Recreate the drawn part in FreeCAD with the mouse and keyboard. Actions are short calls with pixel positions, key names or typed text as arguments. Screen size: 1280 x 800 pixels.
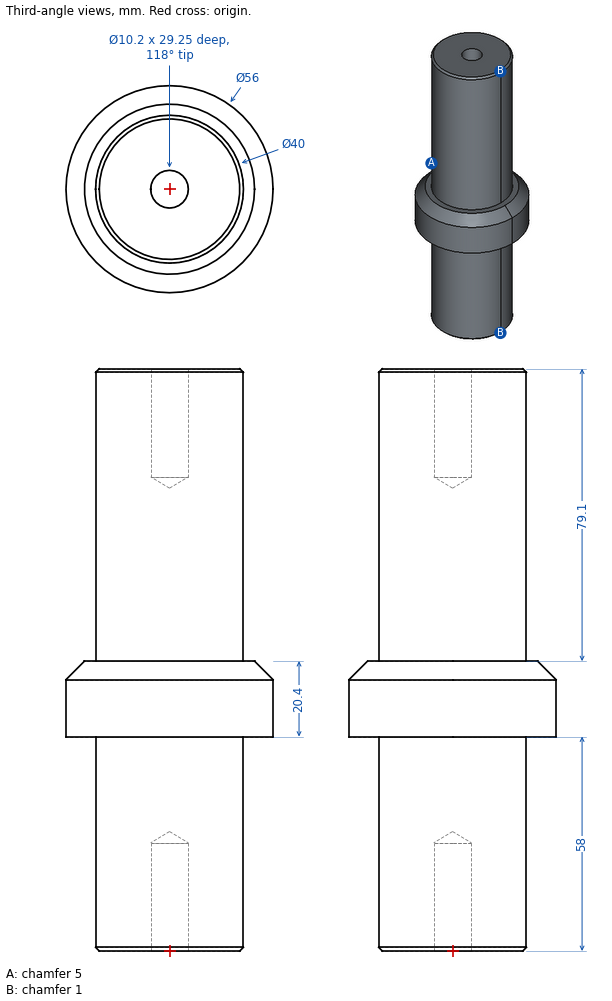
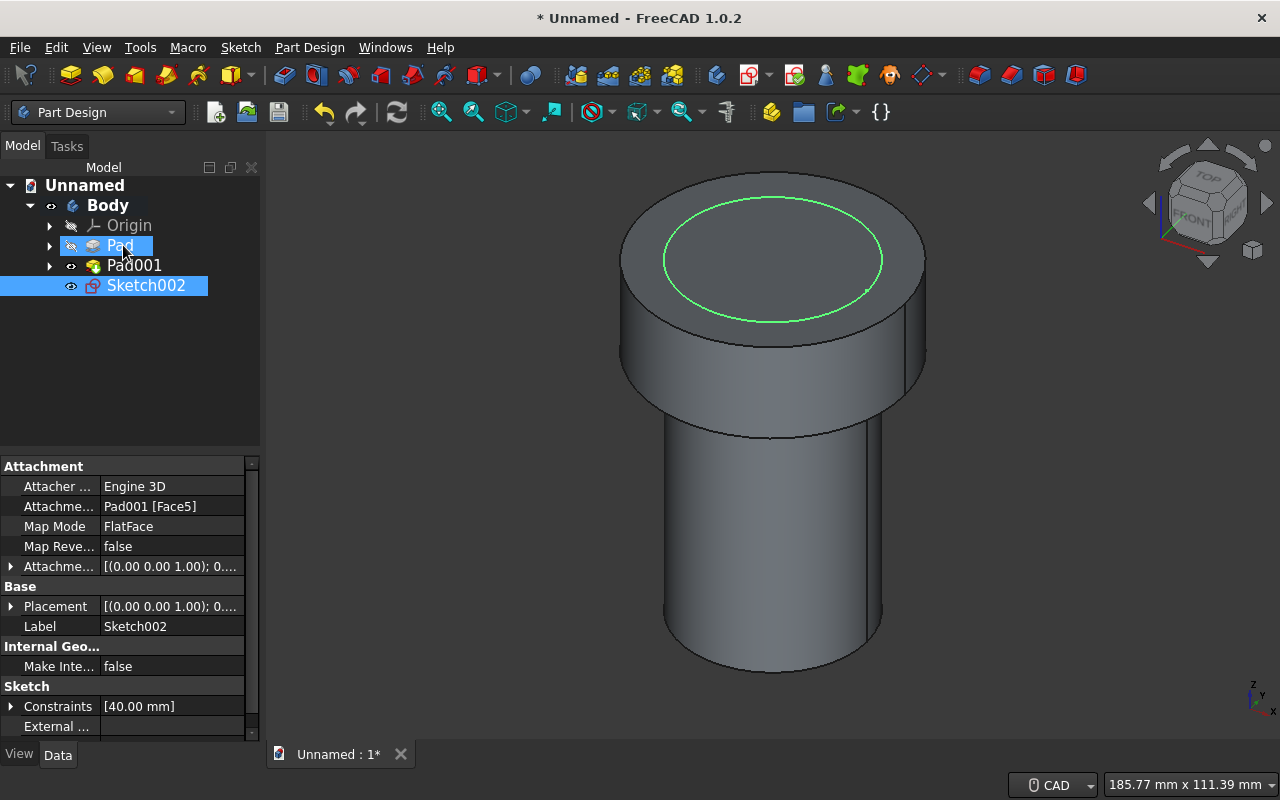
click(72, 76)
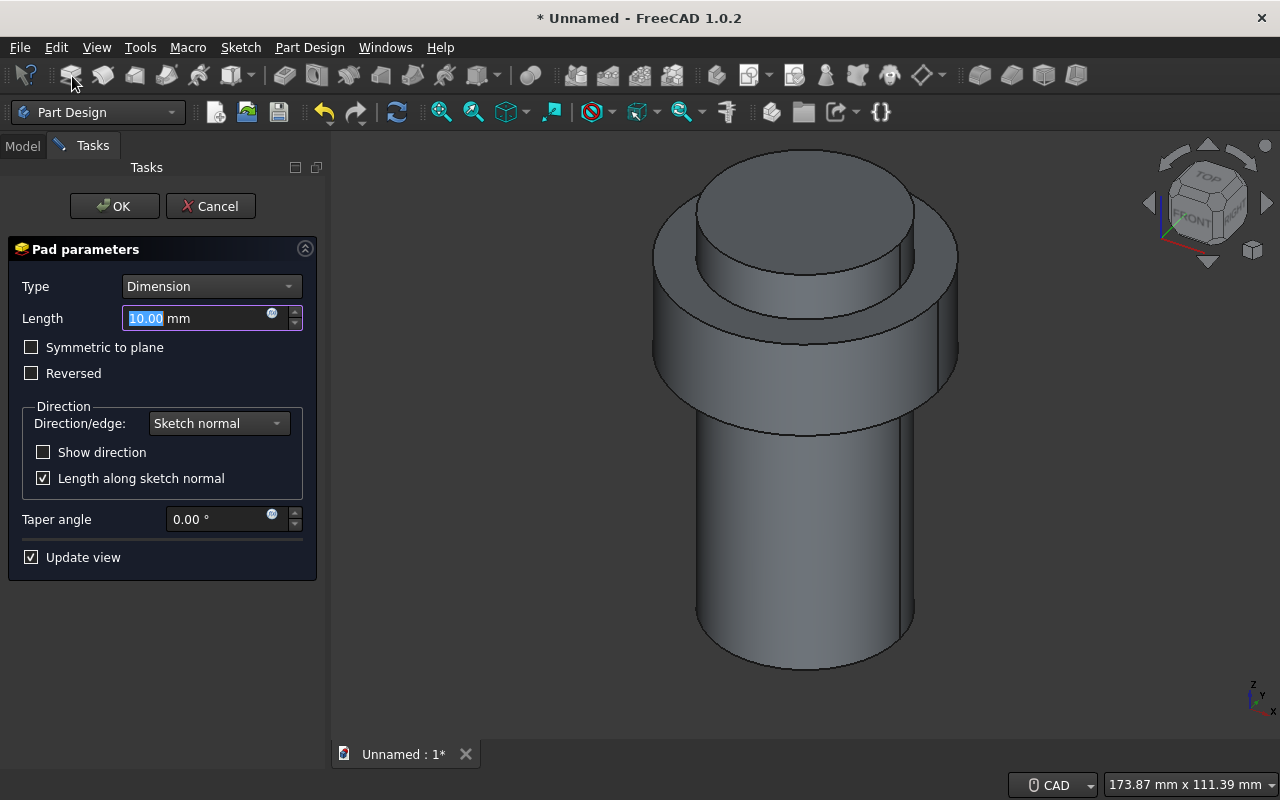
text(79.1)
key(Tab)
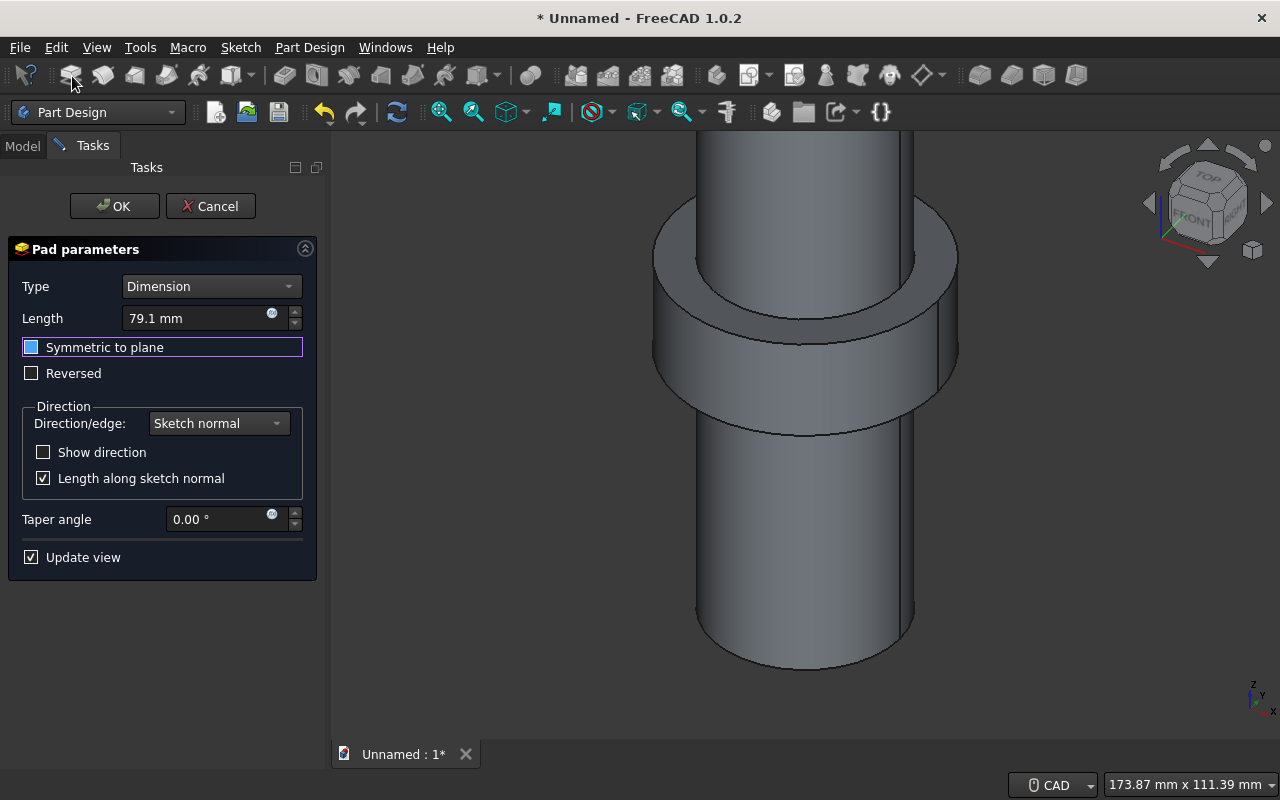
click(115, 206)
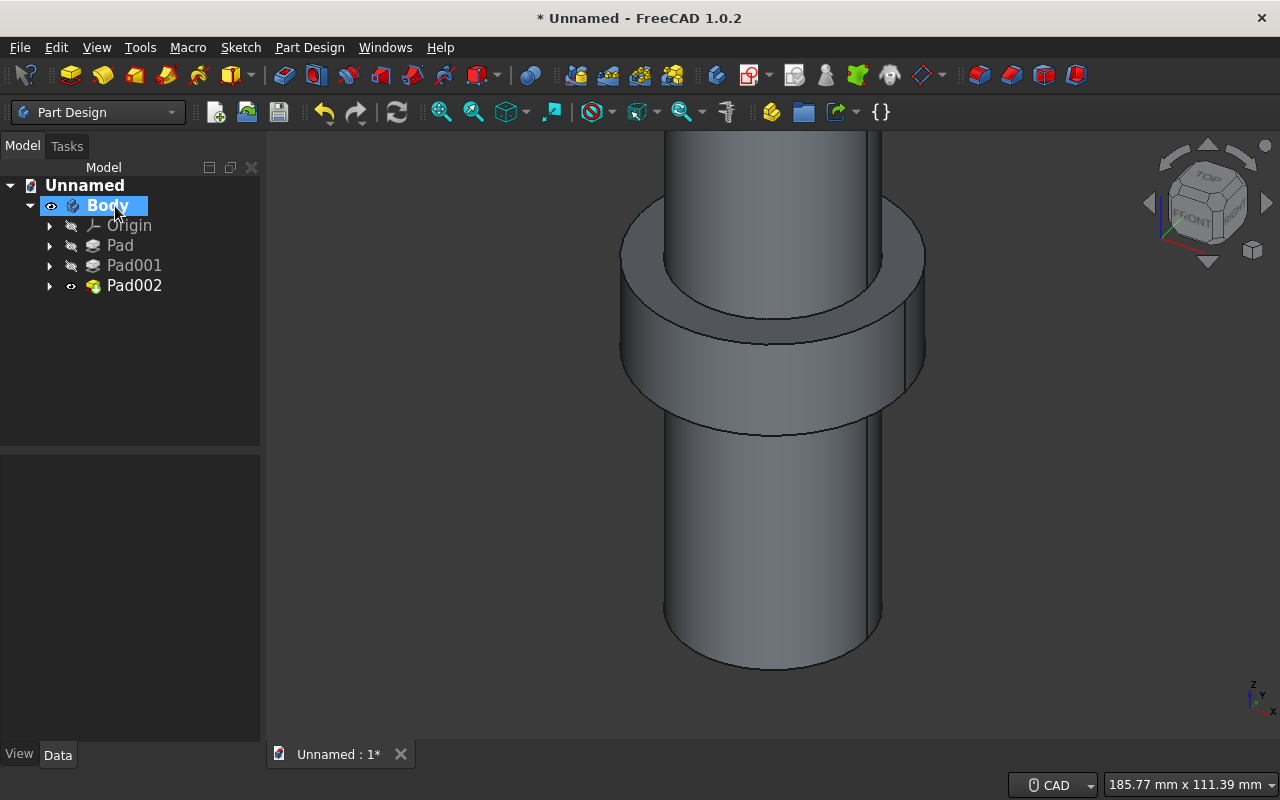
click(442, 112)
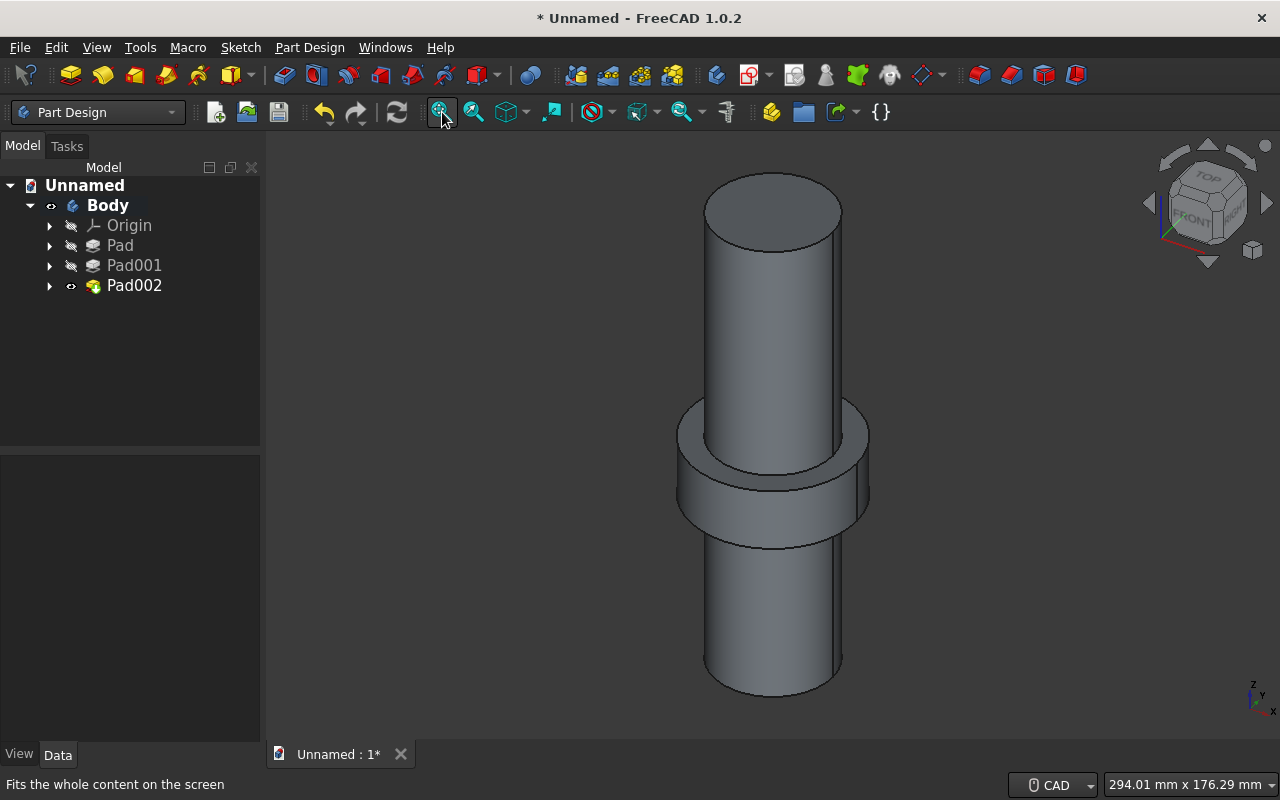
click(677, 441)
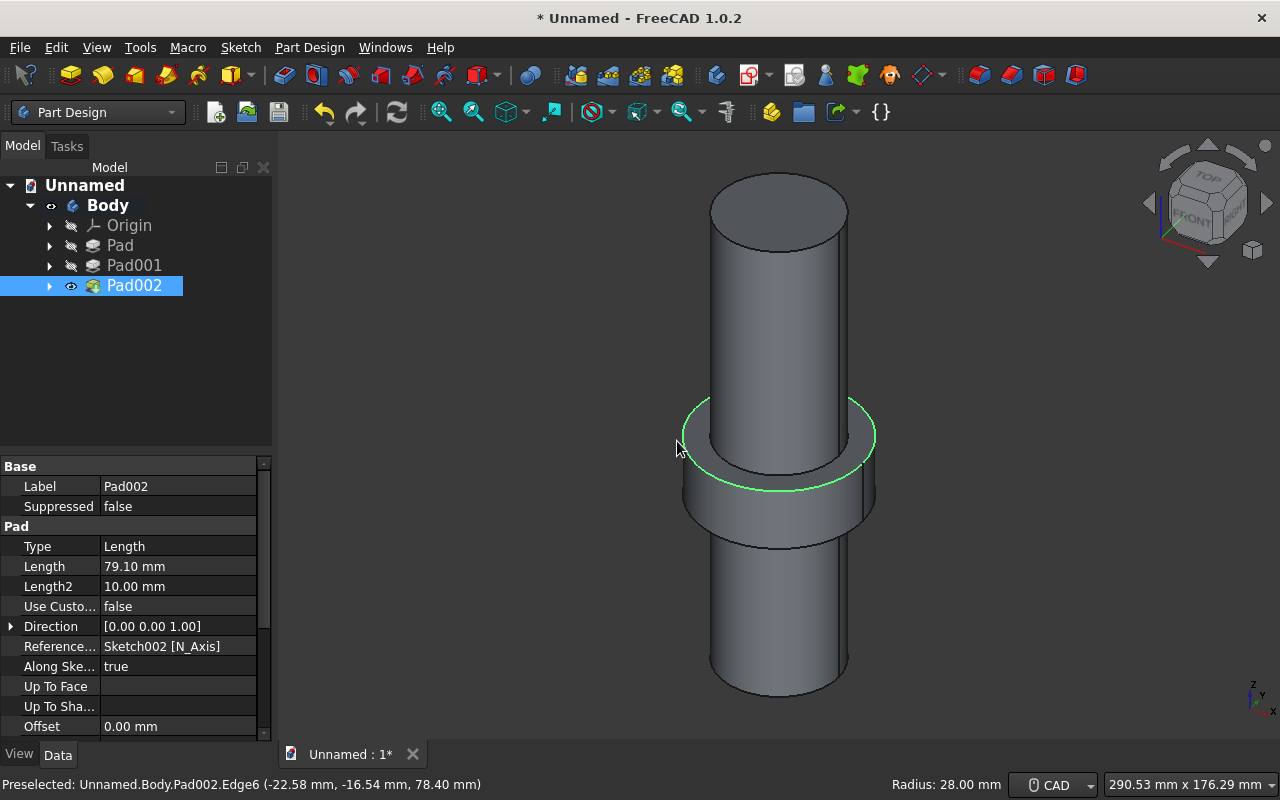
click(1012, 76)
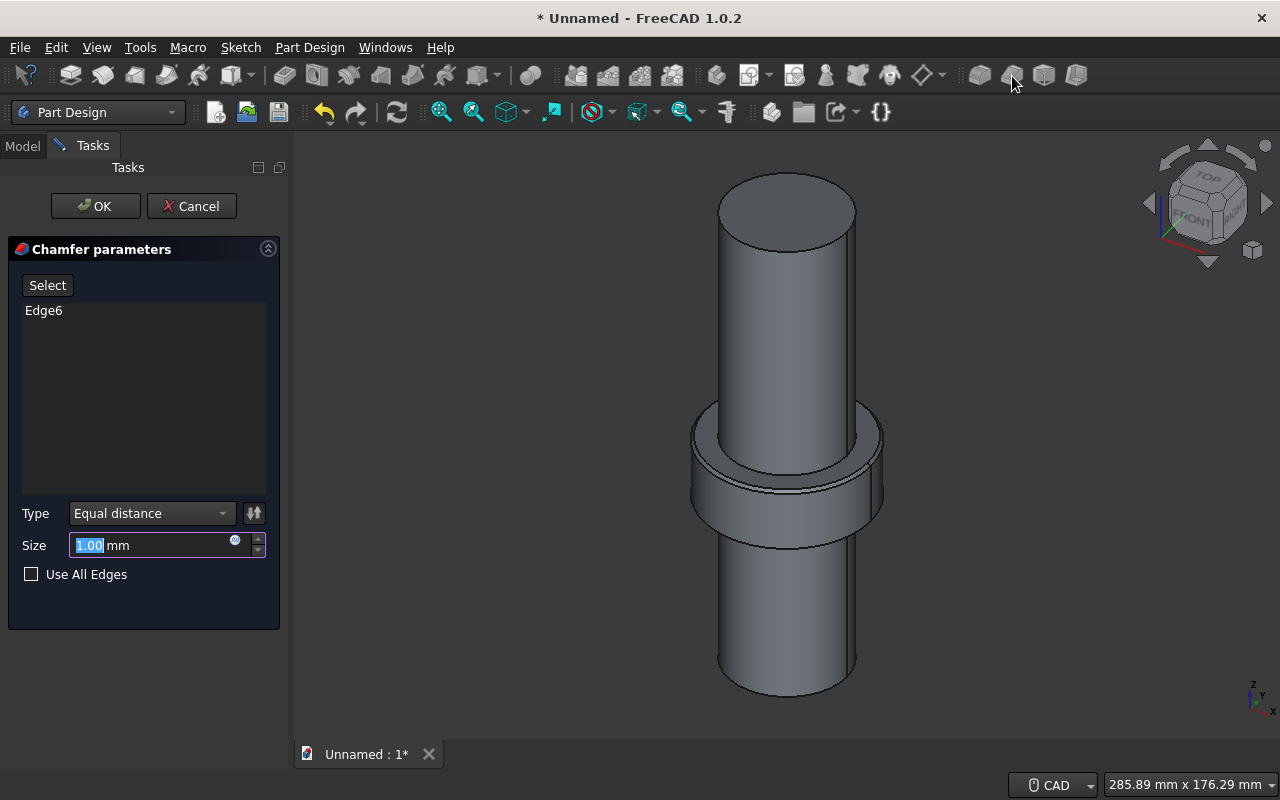
text(5)
key(Tab)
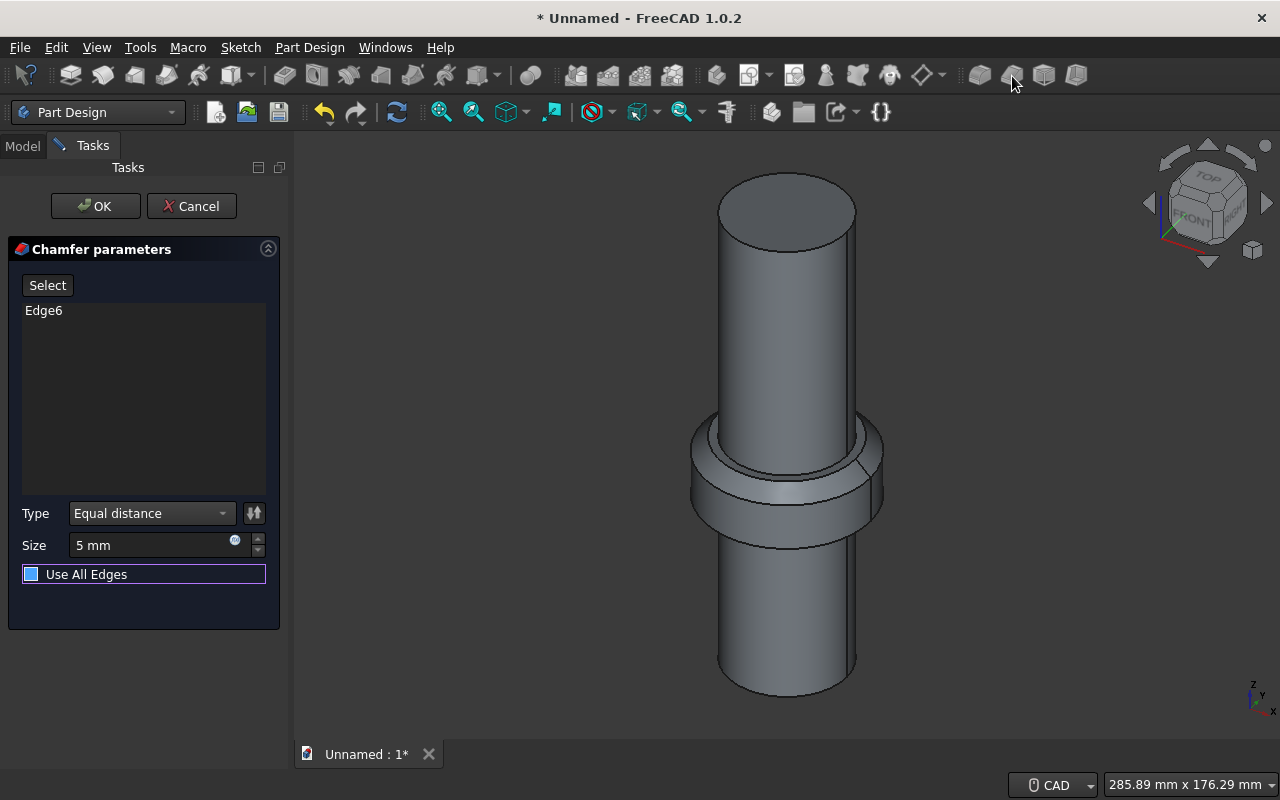
click(96, 206)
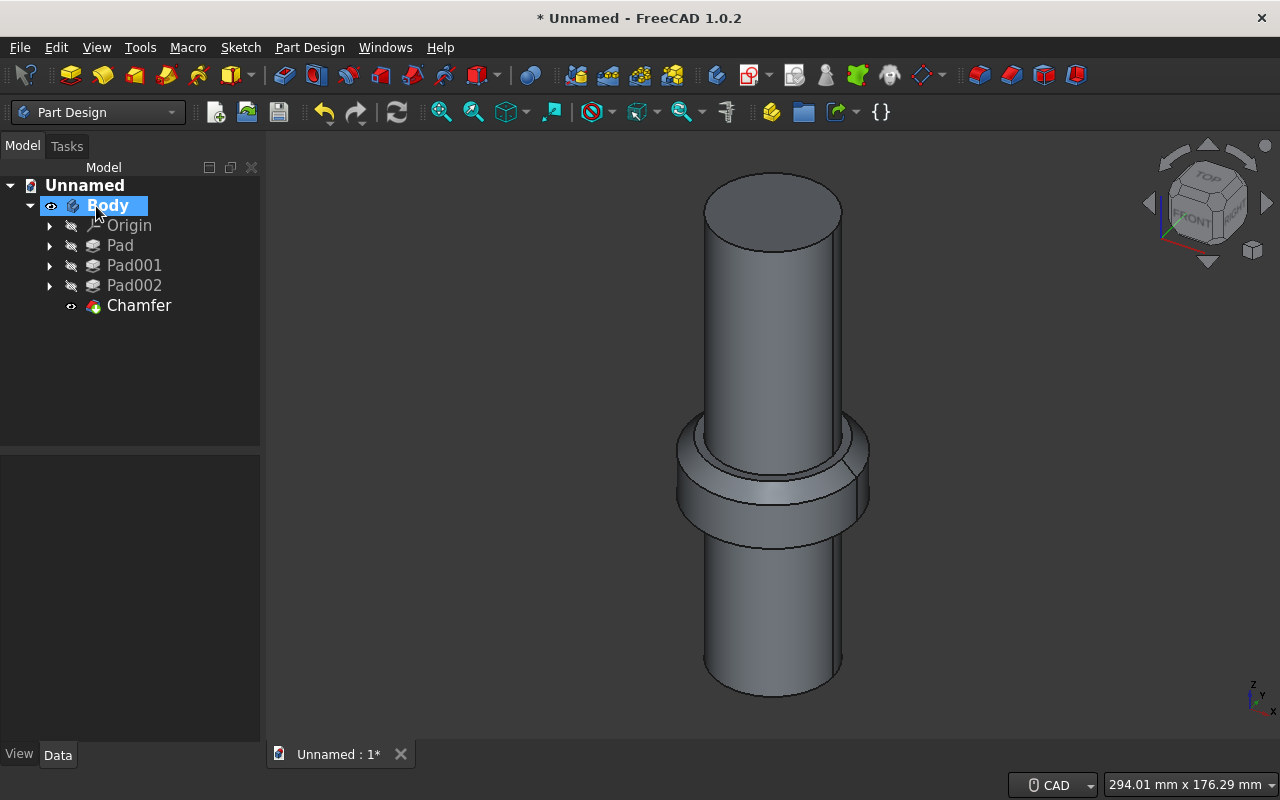
click(704, 216)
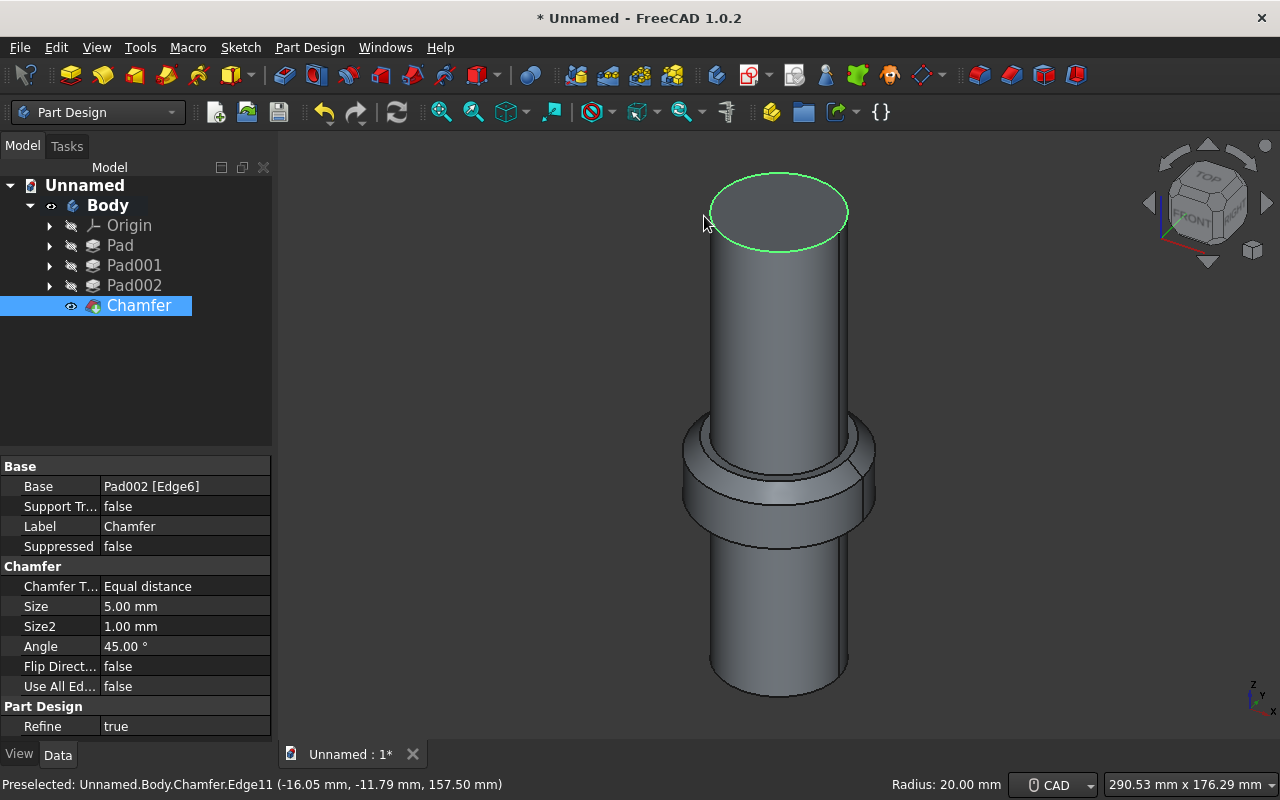
key(0)